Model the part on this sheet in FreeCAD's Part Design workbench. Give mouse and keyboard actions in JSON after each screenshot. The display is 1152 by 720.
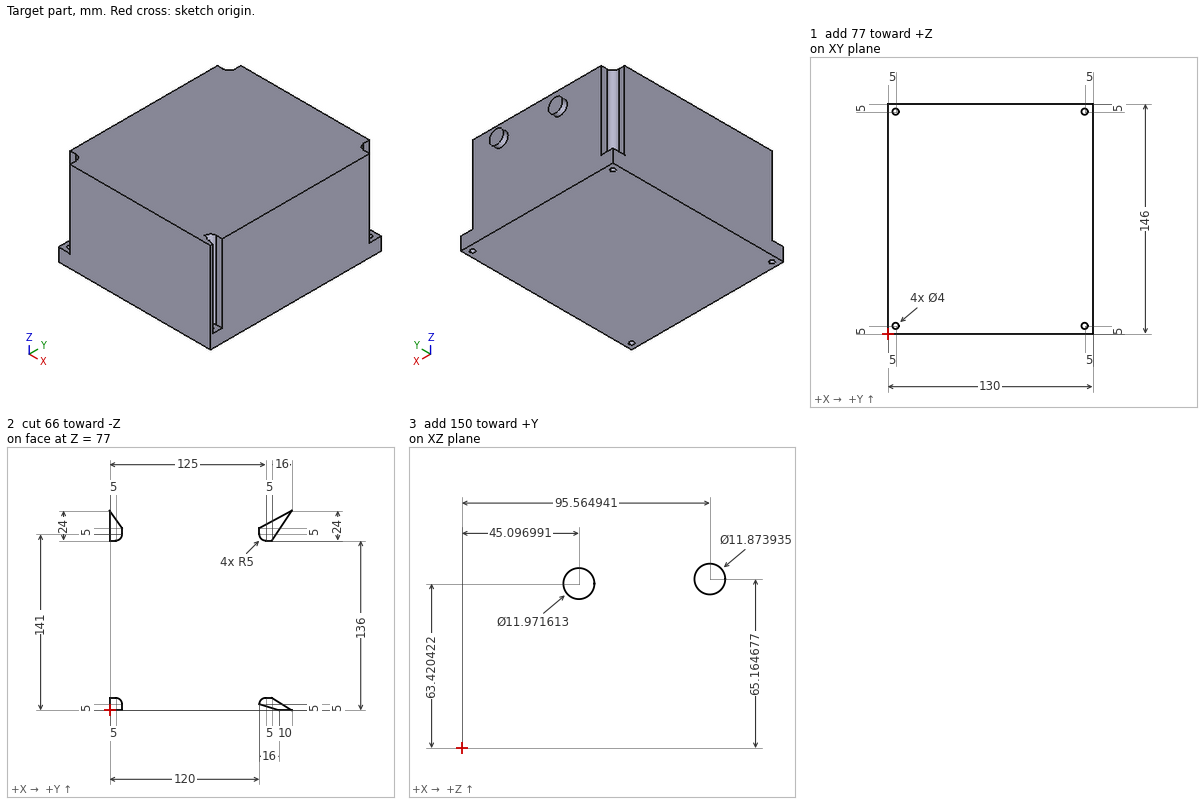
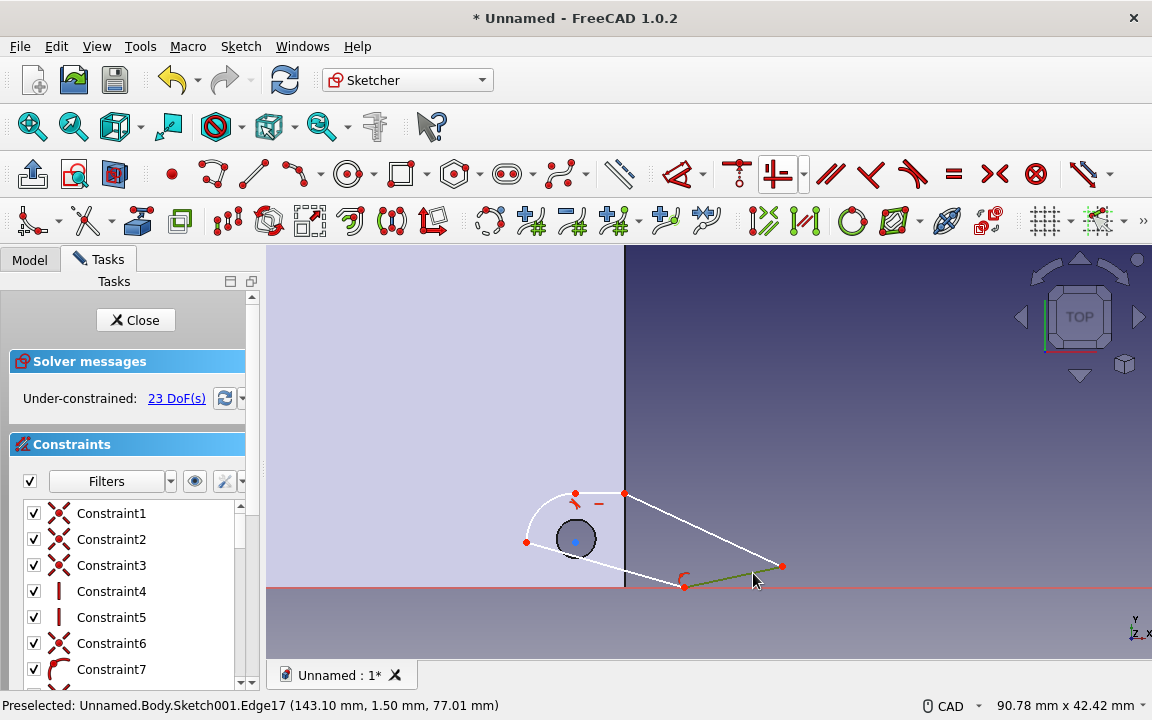
{"action": "key", "text": "h"}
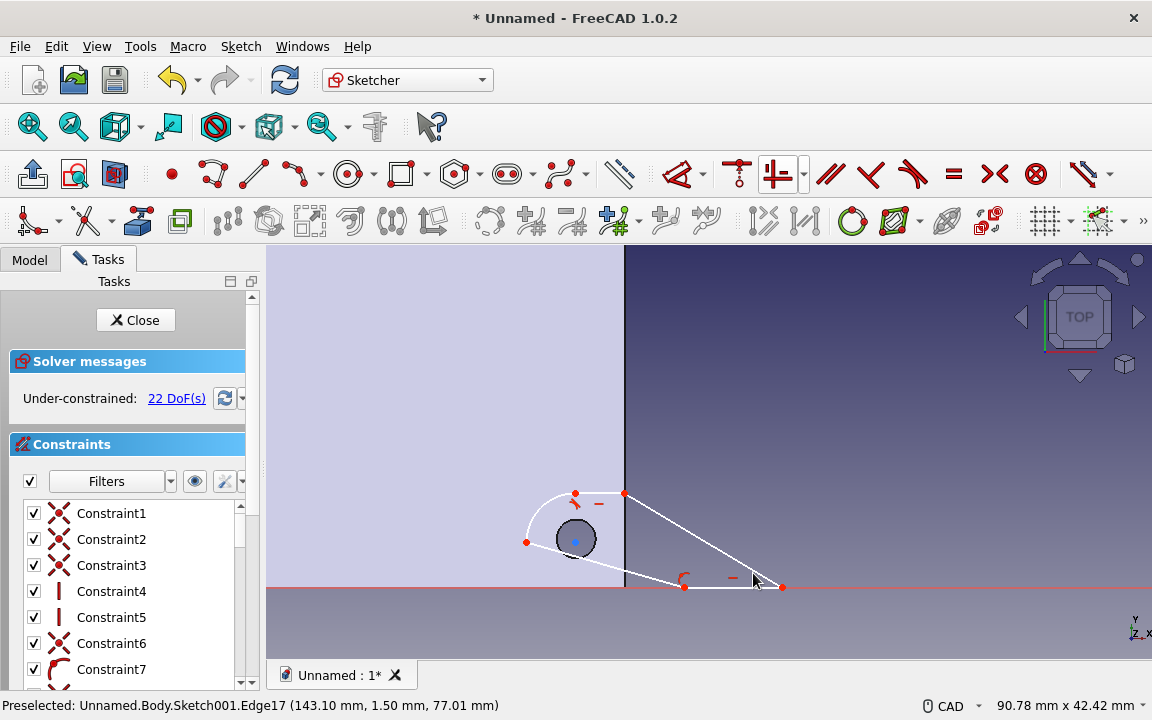
{"action": "scroll", "coordinate": [754, 580], "scroll_direction": "down", "scroll_amount": 9}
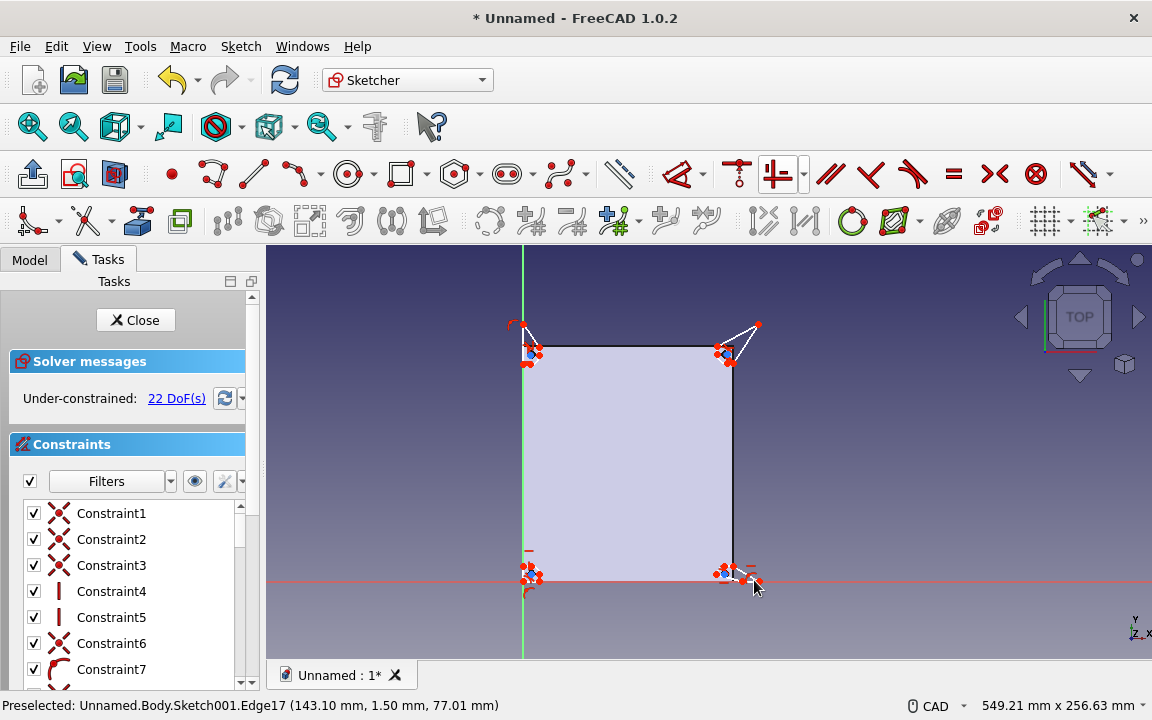
{"action": "scroll", "coordinate": [718, 358], "scroll_direction": "up", "scroll_amount": 6}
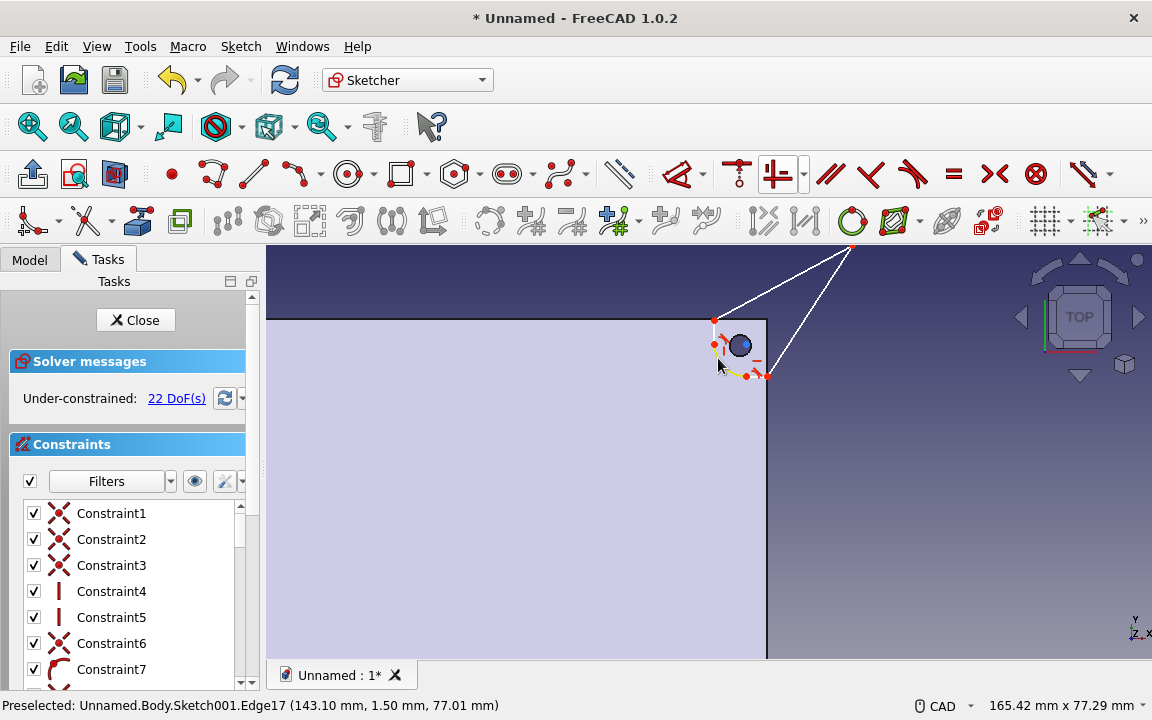
{"action": "left_click", "coordinate": [718, 359]}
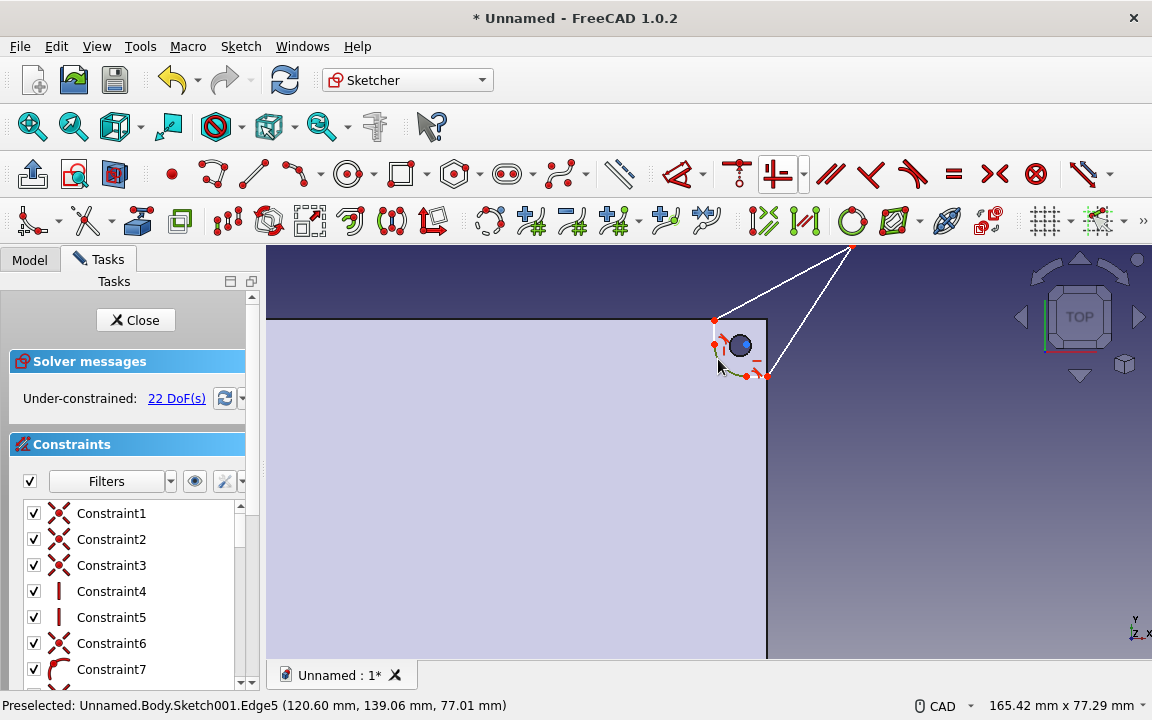
{"action": "scroll", "coordinate": [718, 357], "scroll_direction": "down", "scroll_amount": 6}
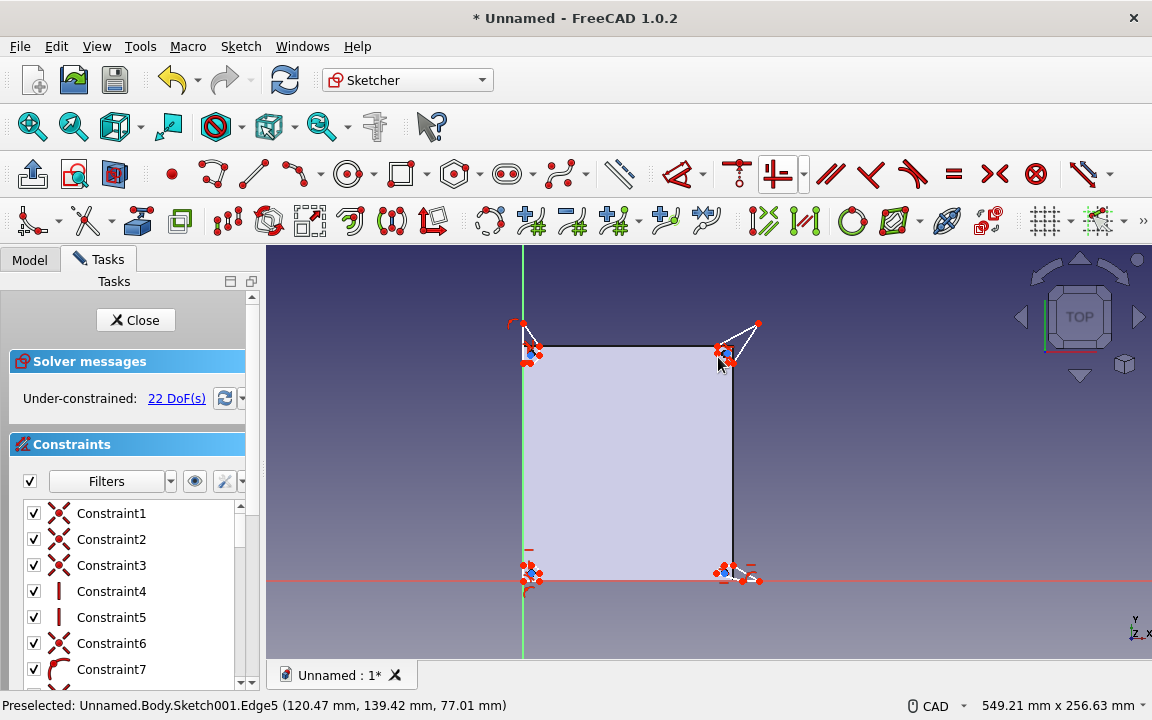
{"action": "scroll", "coordinate": [534, 363], "scroll_direction": "up", "scroll_amount": 7}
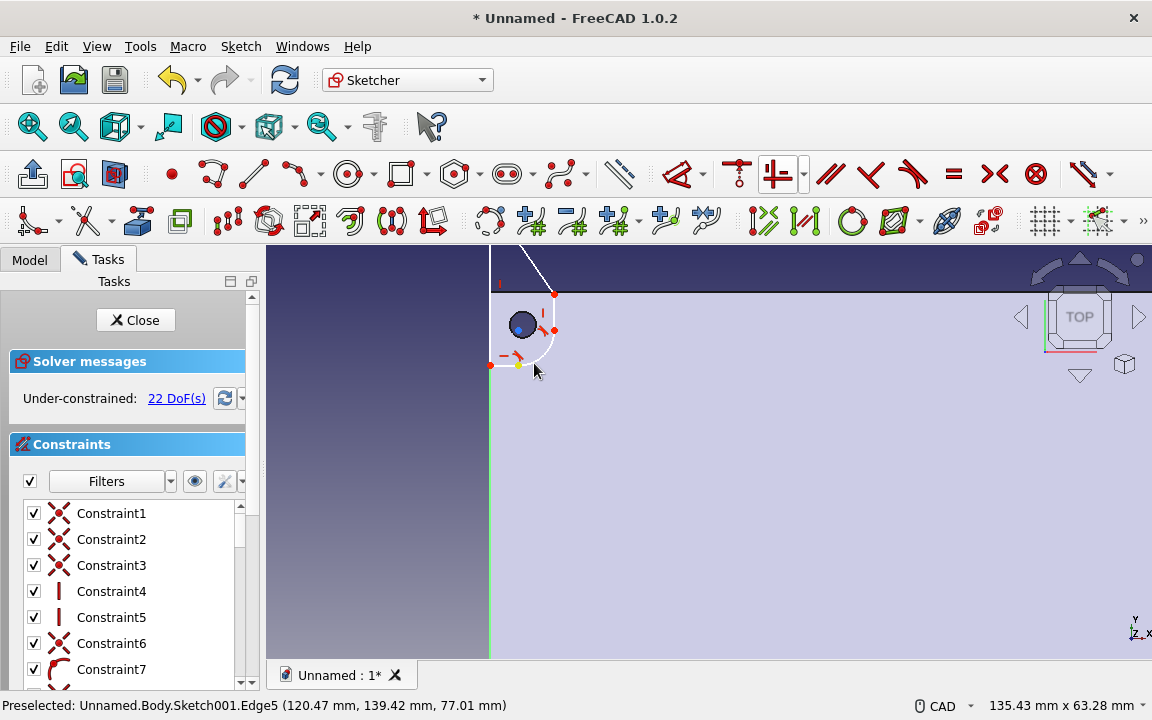
{"action": "left_click", "coordinate": [535, 362]}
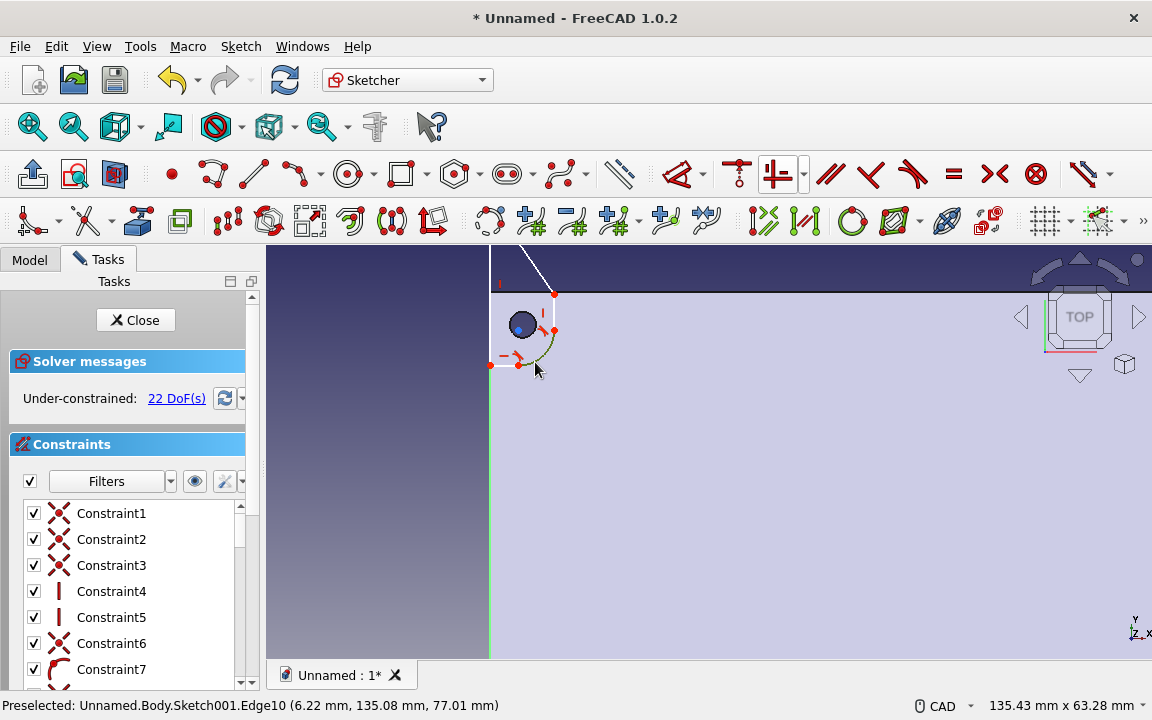
{"action": "scroll", "coordinate": [533, 363], "scroll_direction": "down", "scroll_amount": 7}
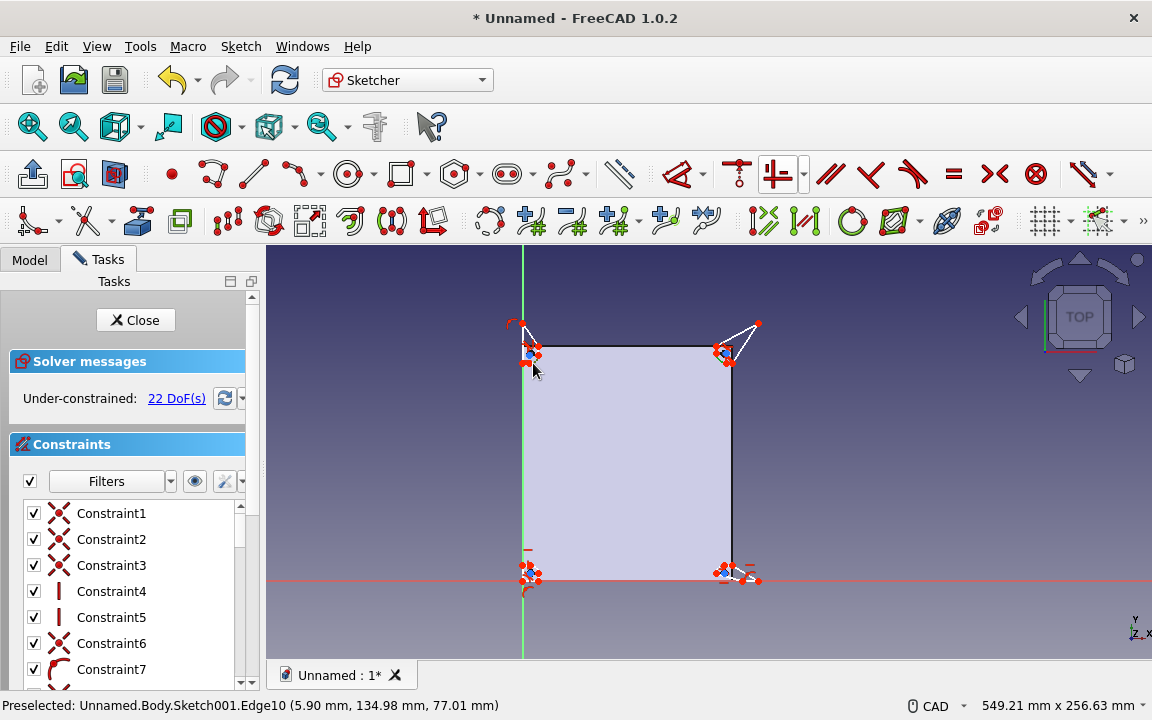
{"action": "scroll", "coordinate": [538, 570], "scroll_direction": "up", "scroll_amount": 7}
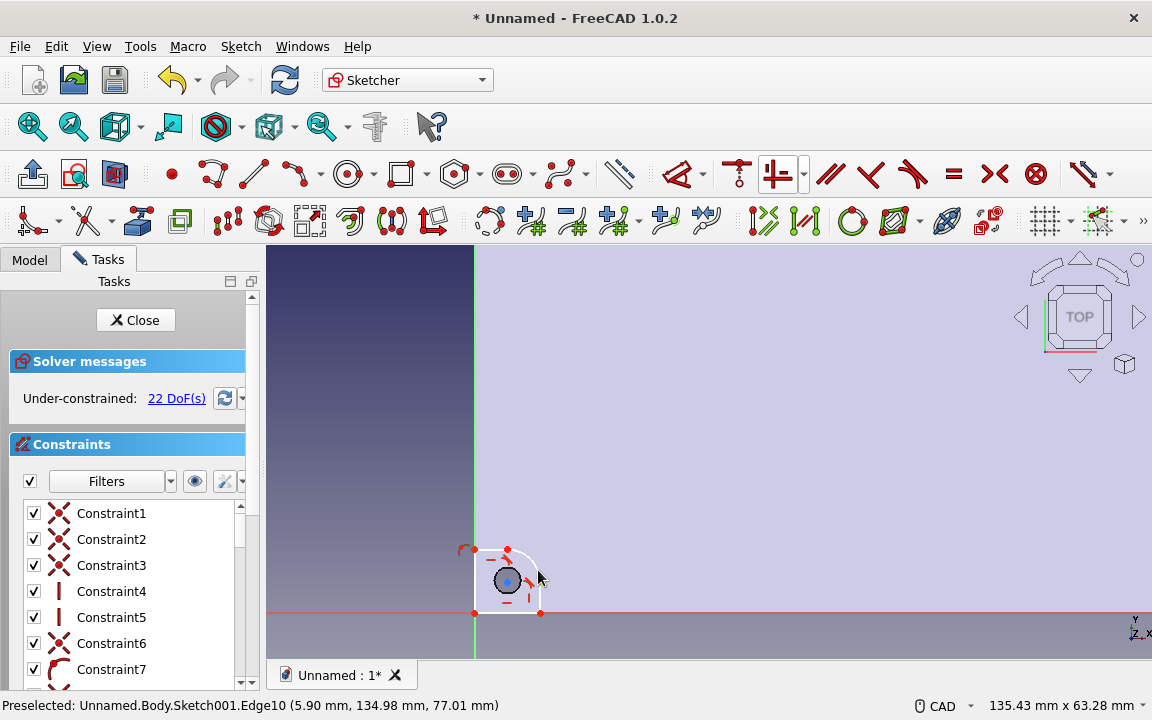
{"action": "left_click", "coordinate": [536, 567]}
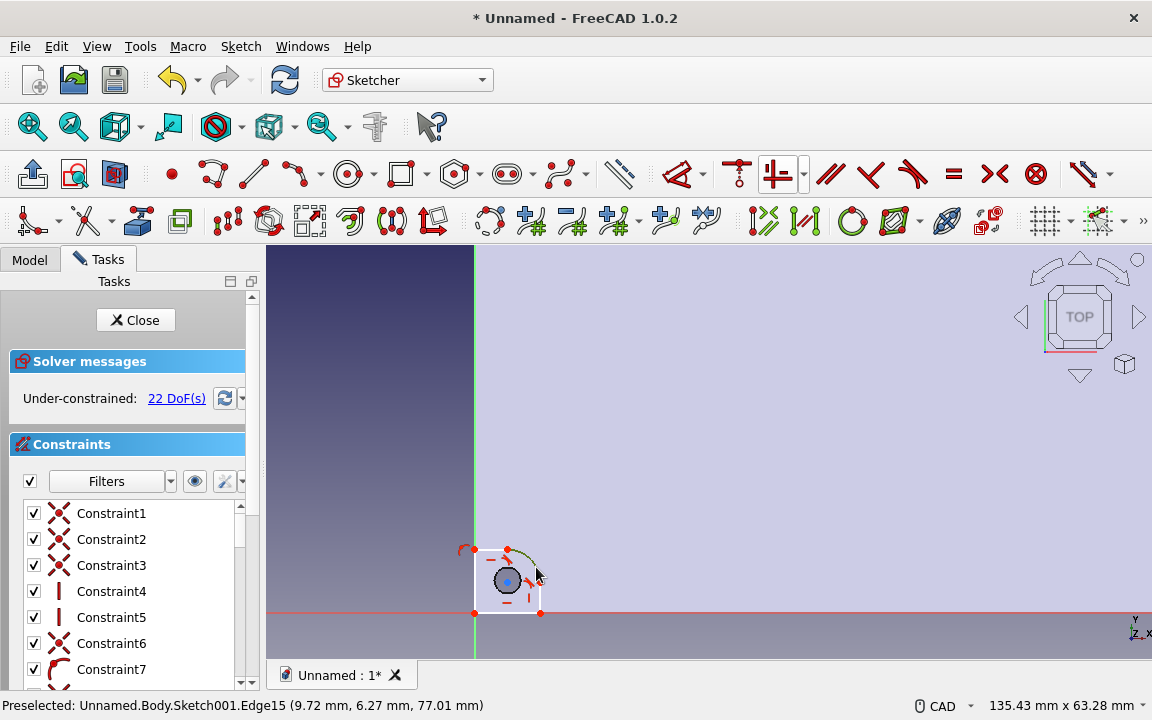
{"action": "scroll", "coordinate": [538, 571], "scroll_direction": "down", "scroll_amount": 7}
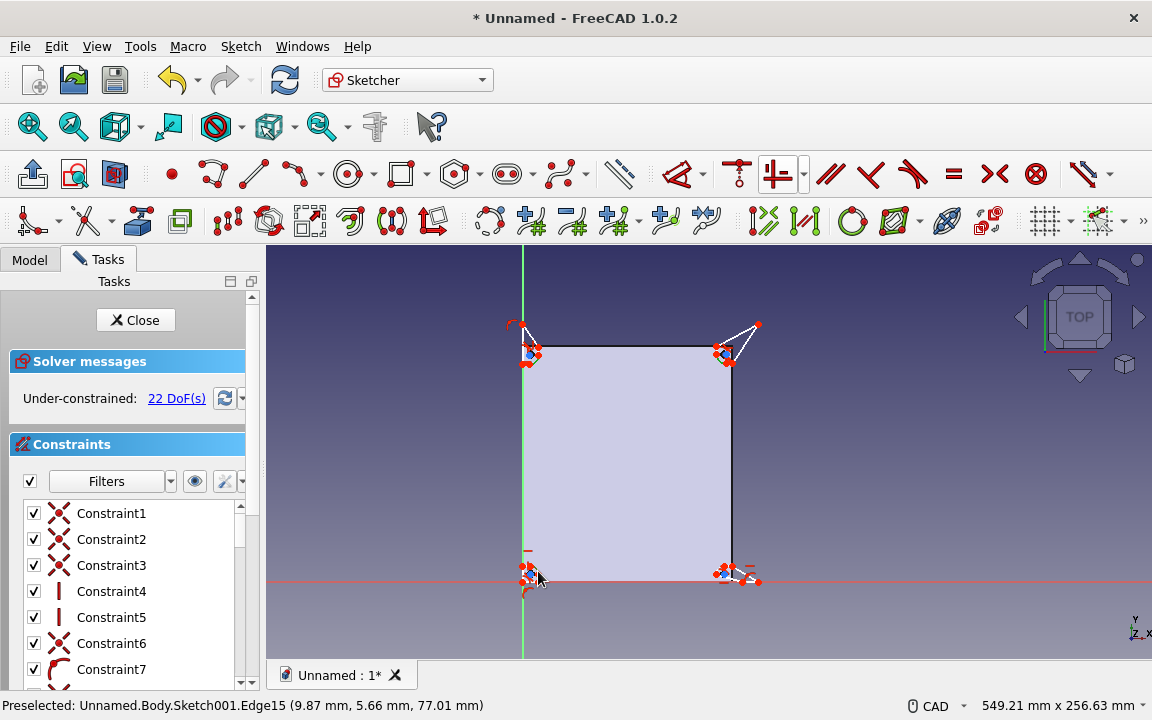
{"action": "scroll", "coordinate": [721, 567], "scroll_direction": "up", "scroll_amount": 7}